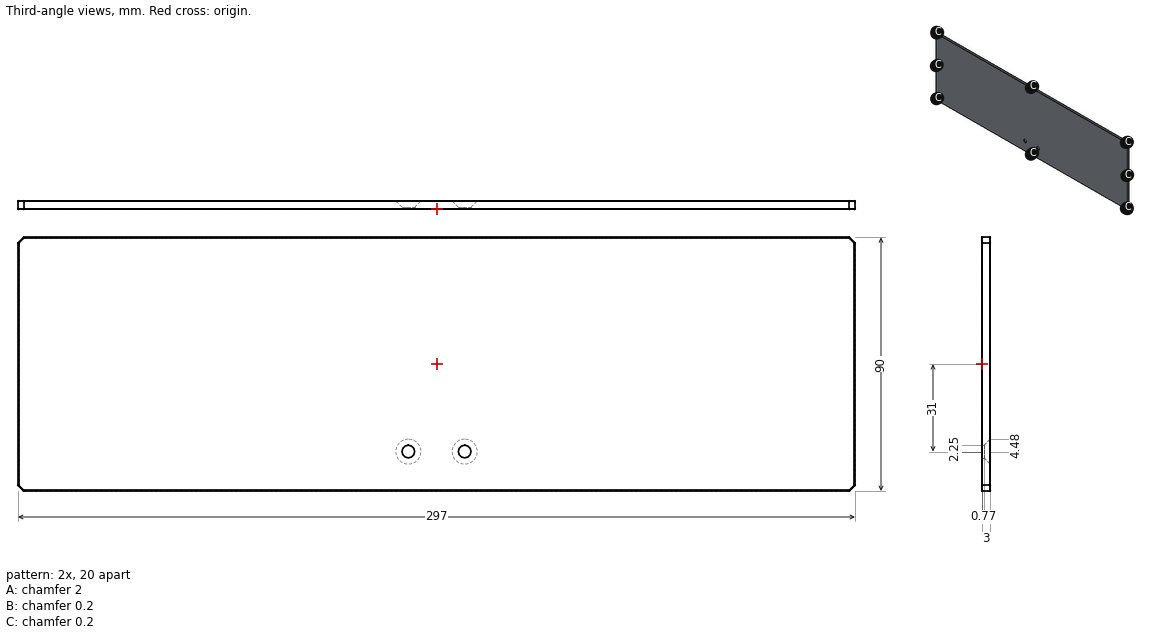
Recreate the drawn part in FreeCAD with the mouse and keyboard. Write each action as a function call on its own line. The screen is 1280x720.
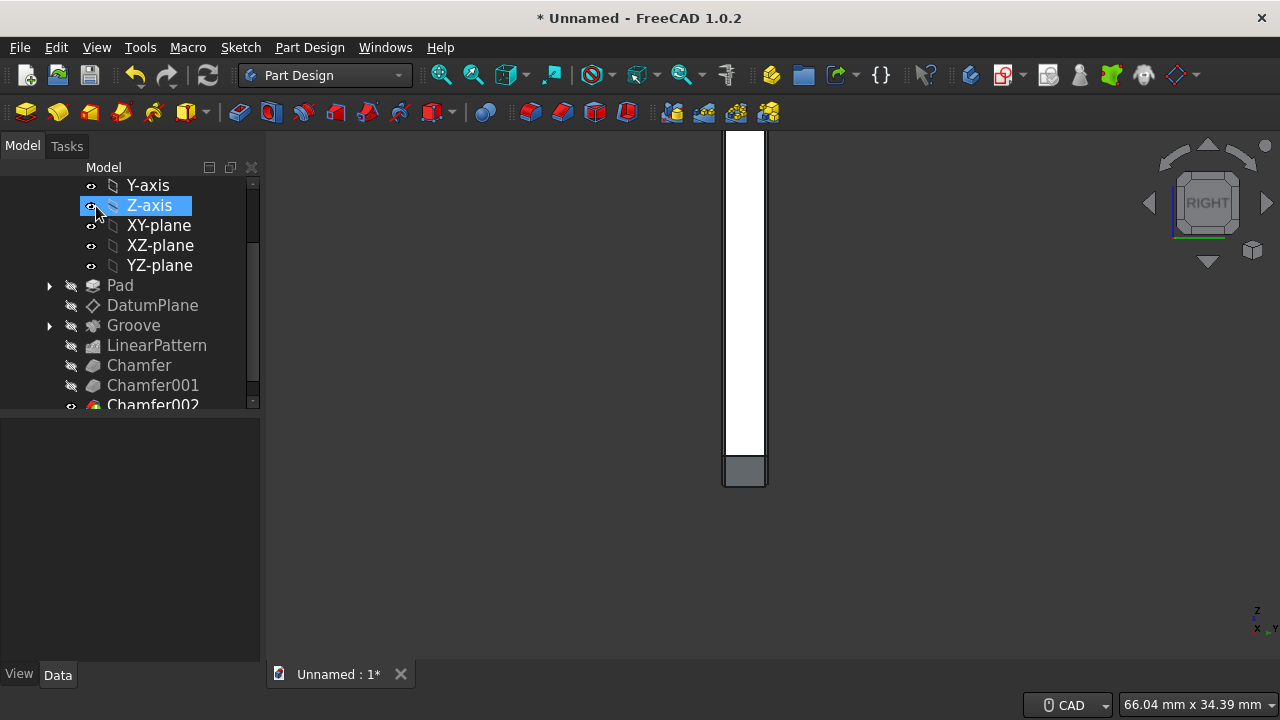
key(0)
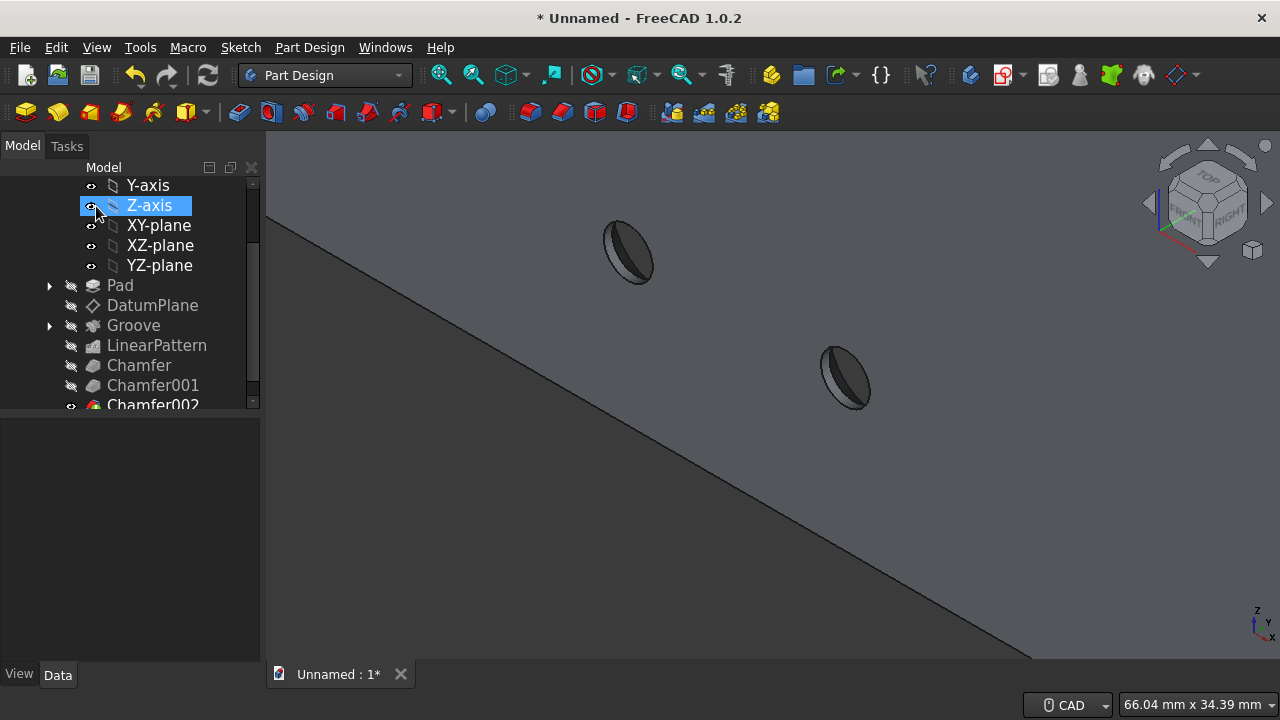
key(v)
key(f)